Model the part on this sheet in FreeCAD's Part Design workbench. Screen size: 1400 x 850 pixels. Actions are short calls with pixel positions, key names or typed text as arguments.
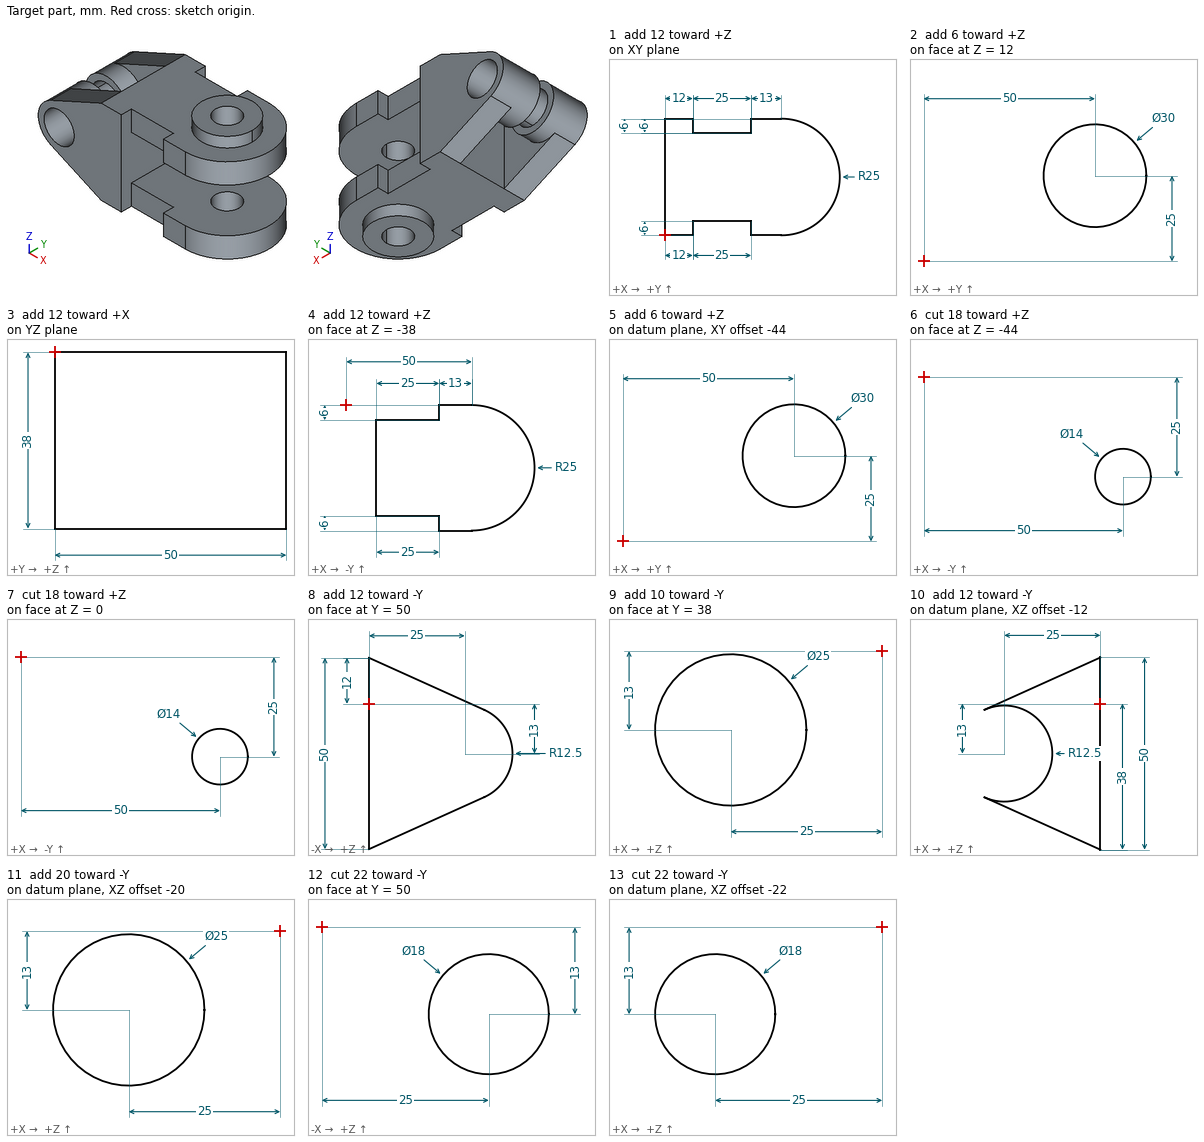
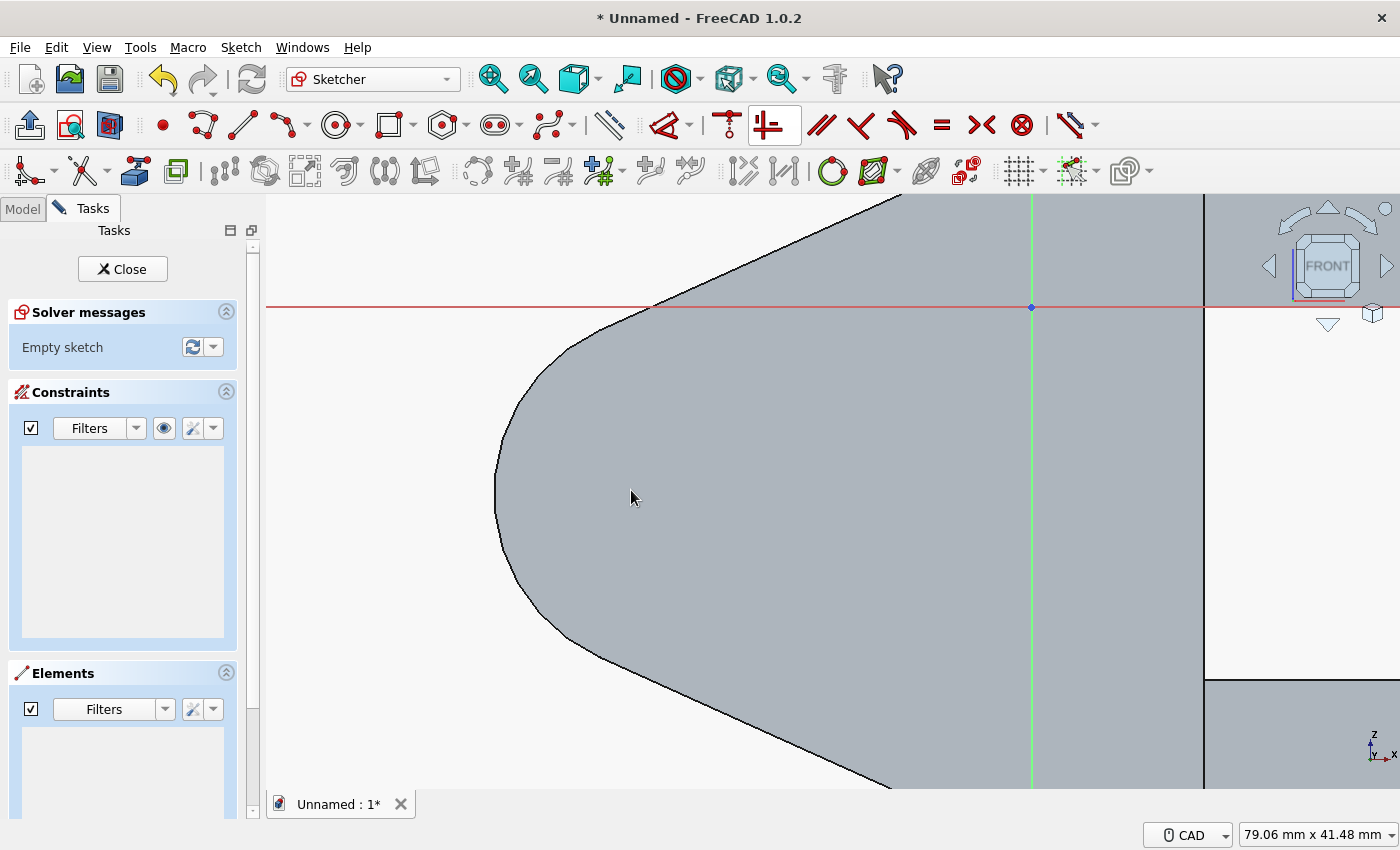
click(336, 126)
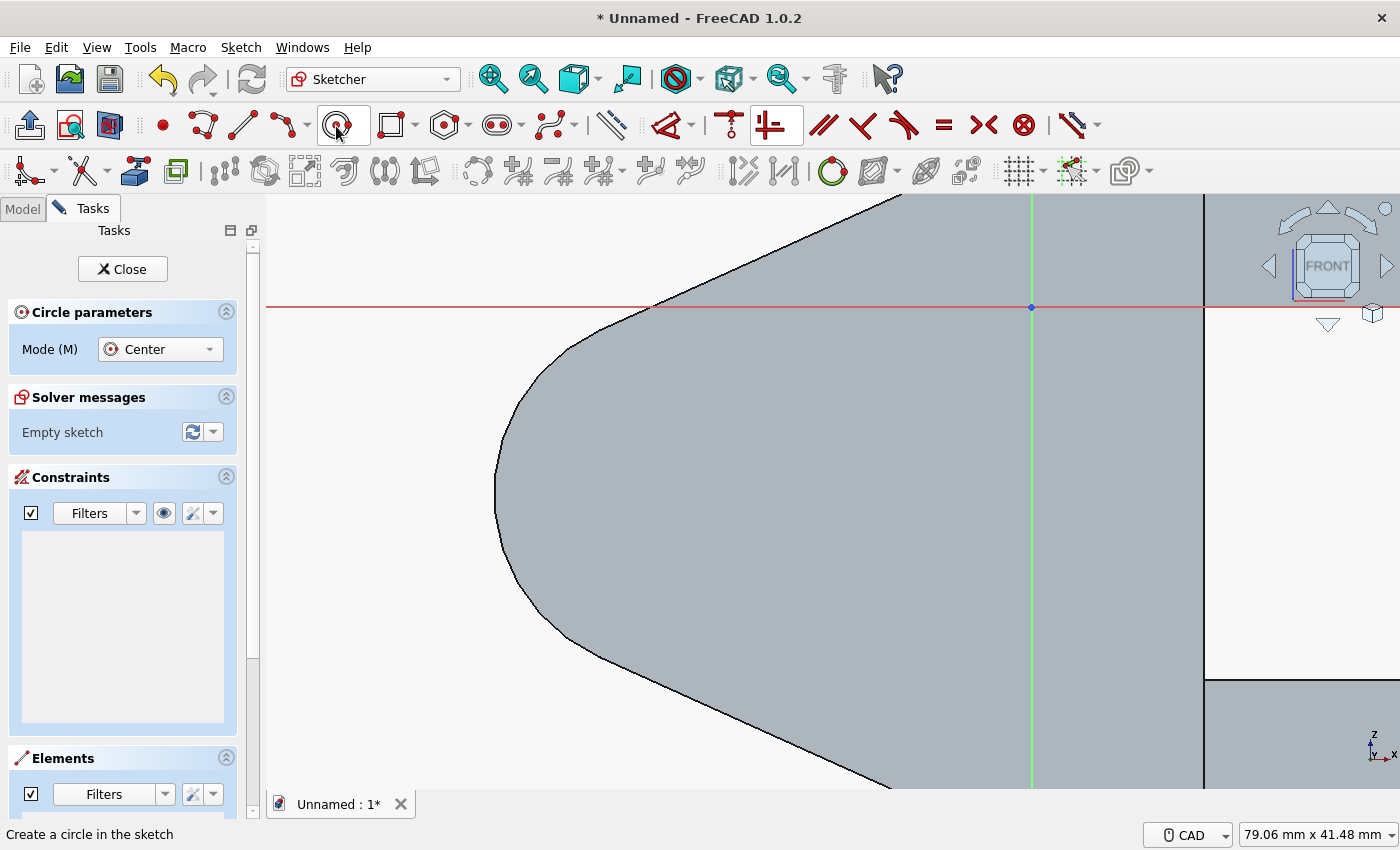
click(673, 494)
click(800, 367)
key(Escape)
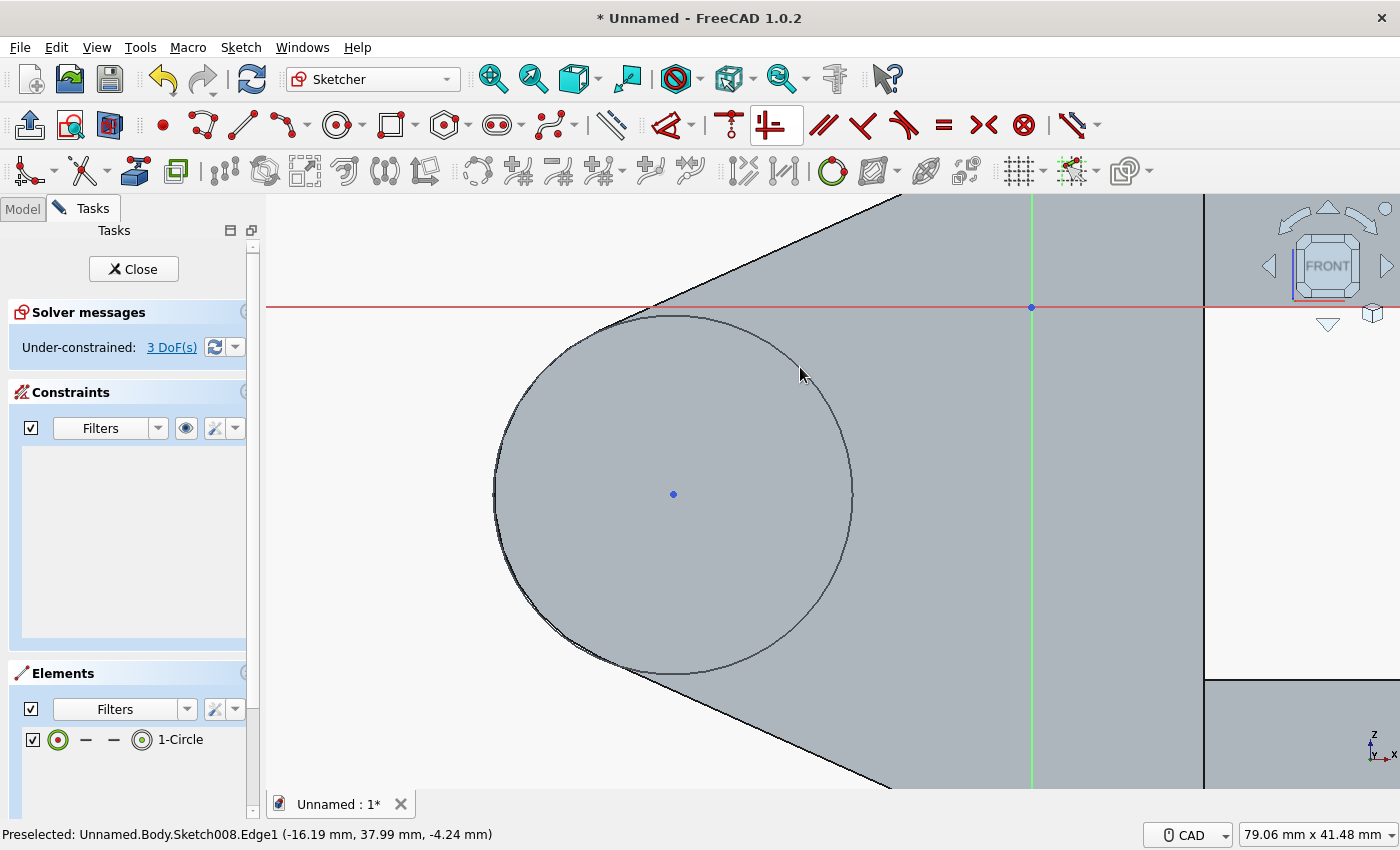
click(666, 126)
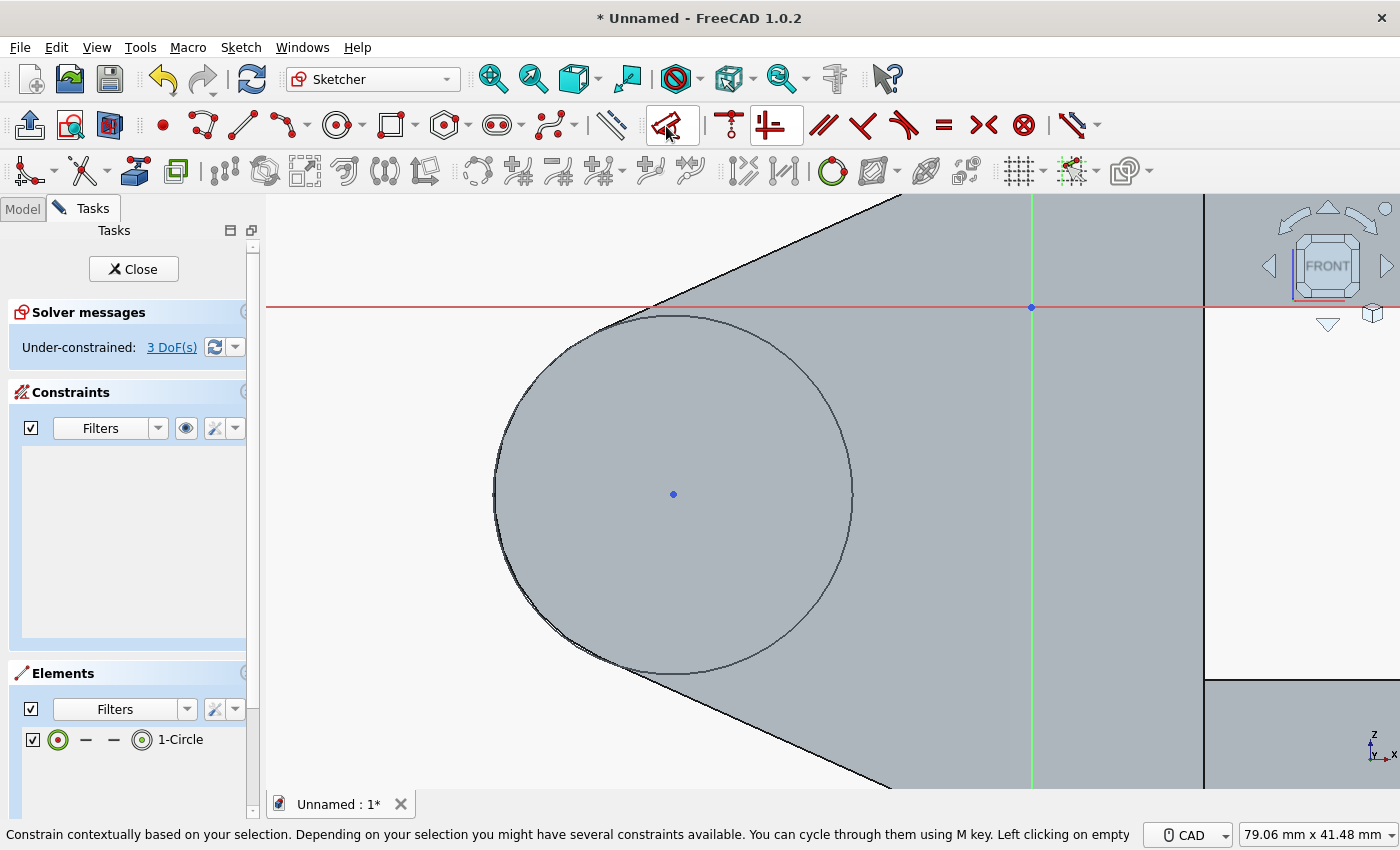
click(800, 368)
click(823, 345)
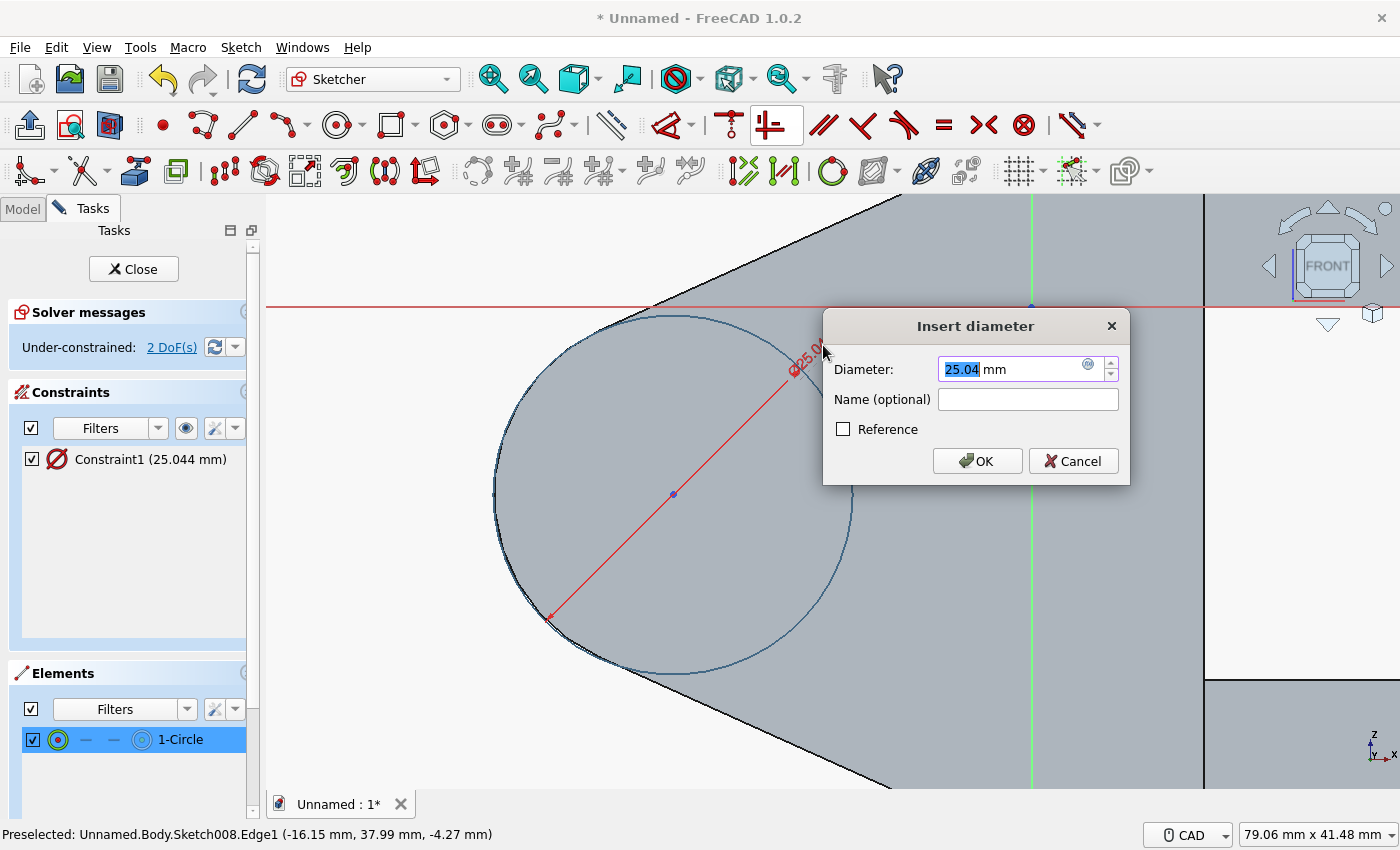
text(25)
key(Return)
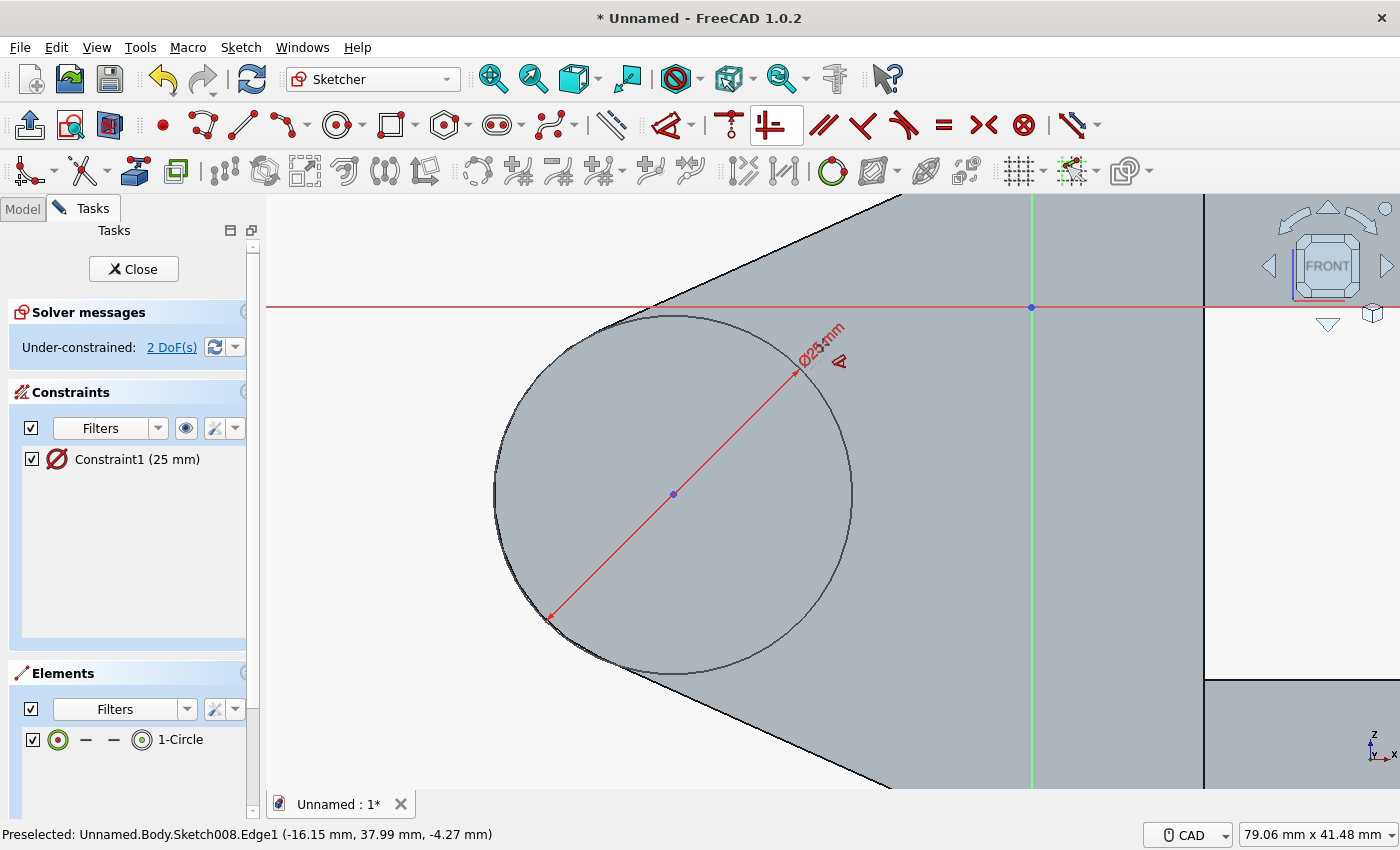
click(673, 495)
click(852, 273)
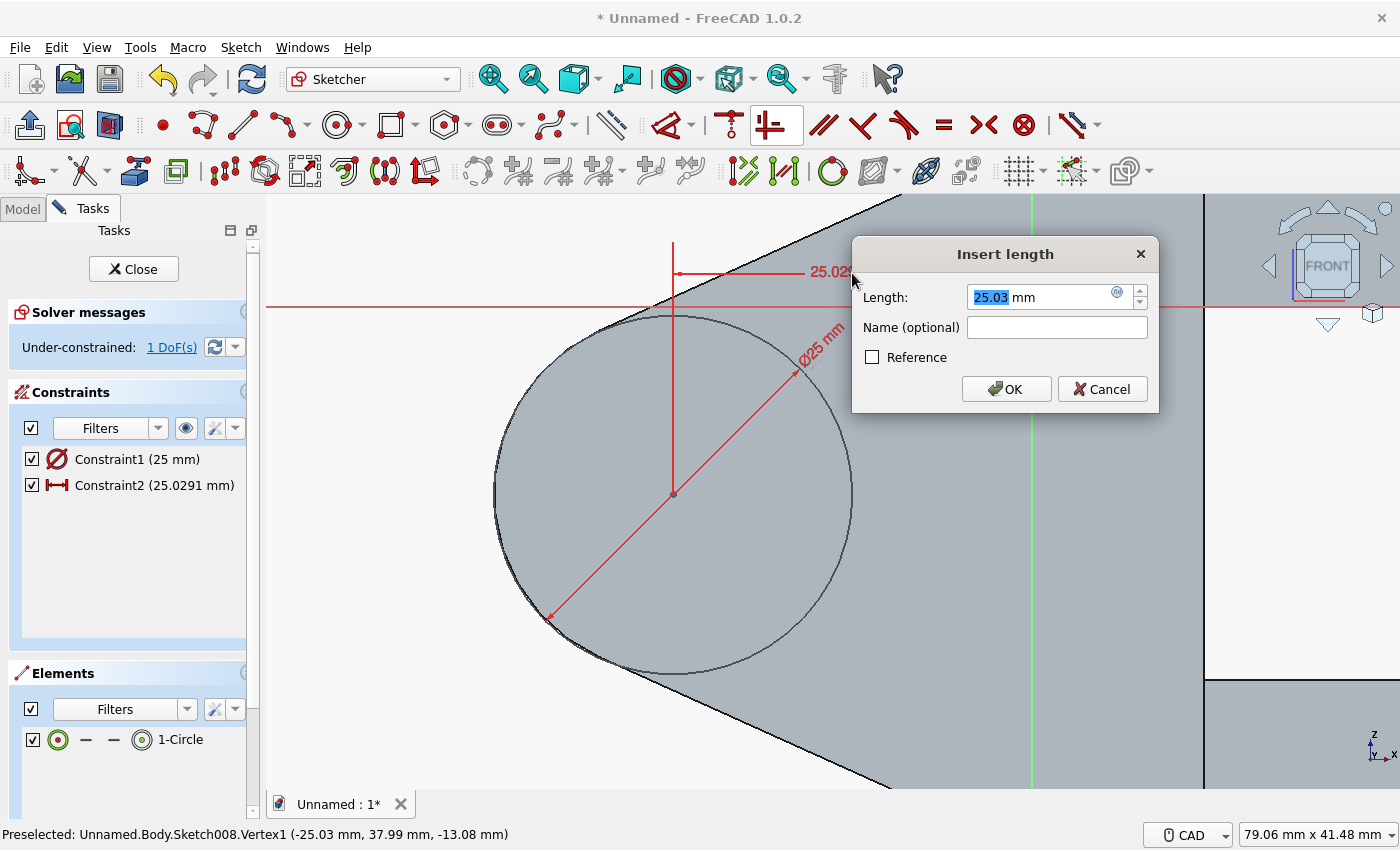
text(25)
key(Return)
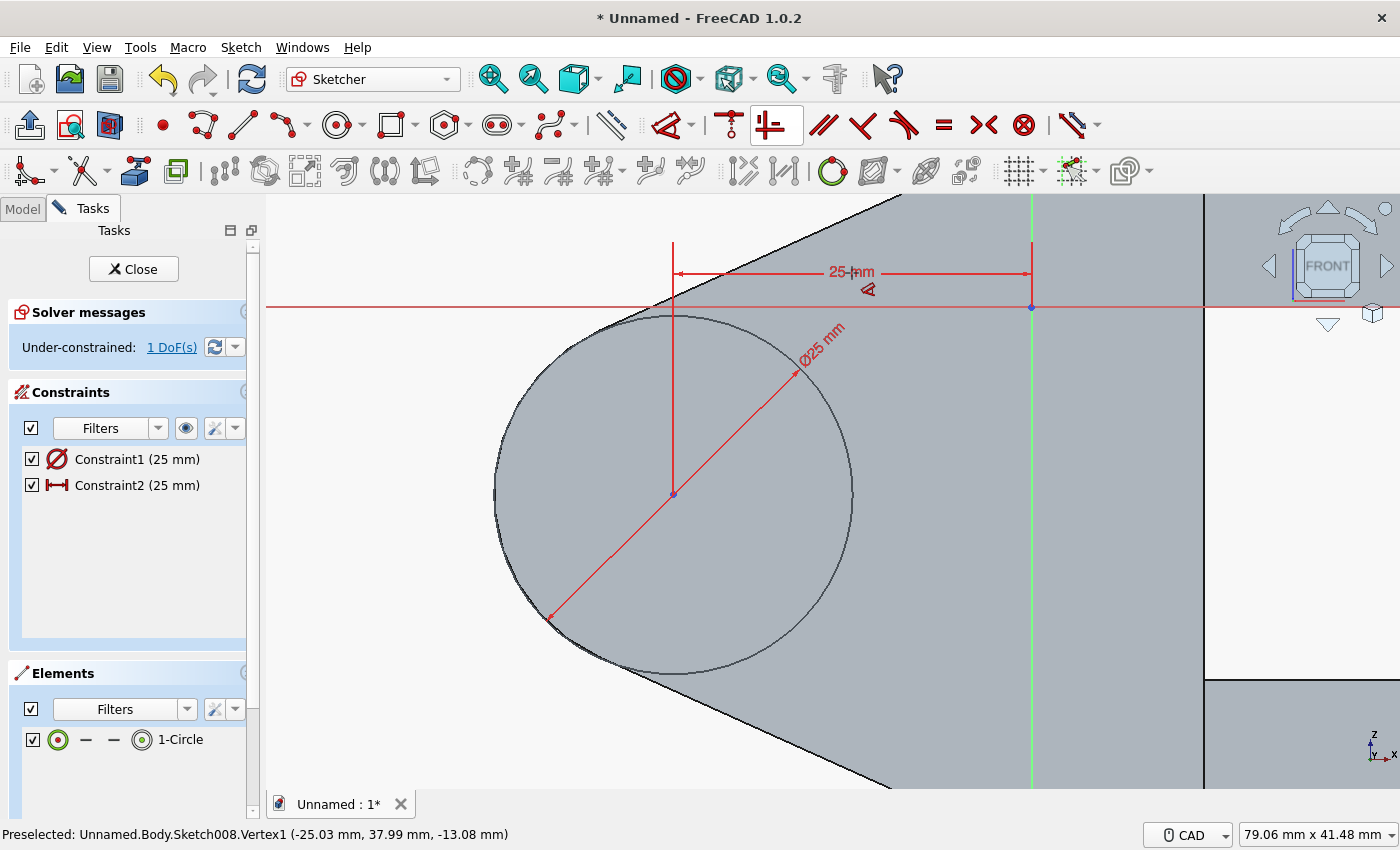
click(673, 495)
click(1066, 401)